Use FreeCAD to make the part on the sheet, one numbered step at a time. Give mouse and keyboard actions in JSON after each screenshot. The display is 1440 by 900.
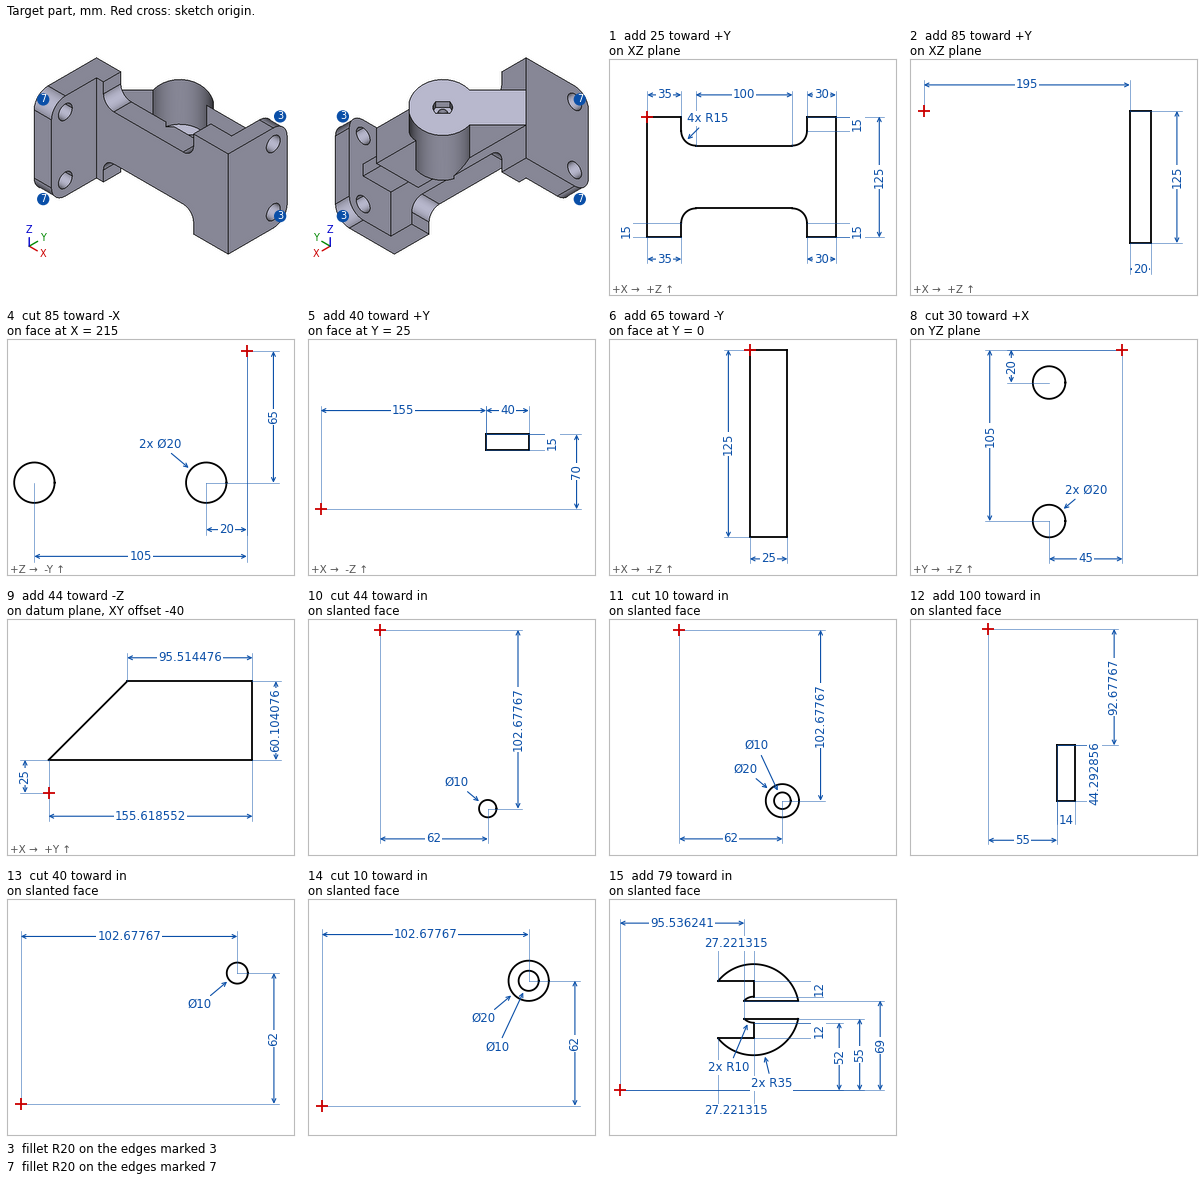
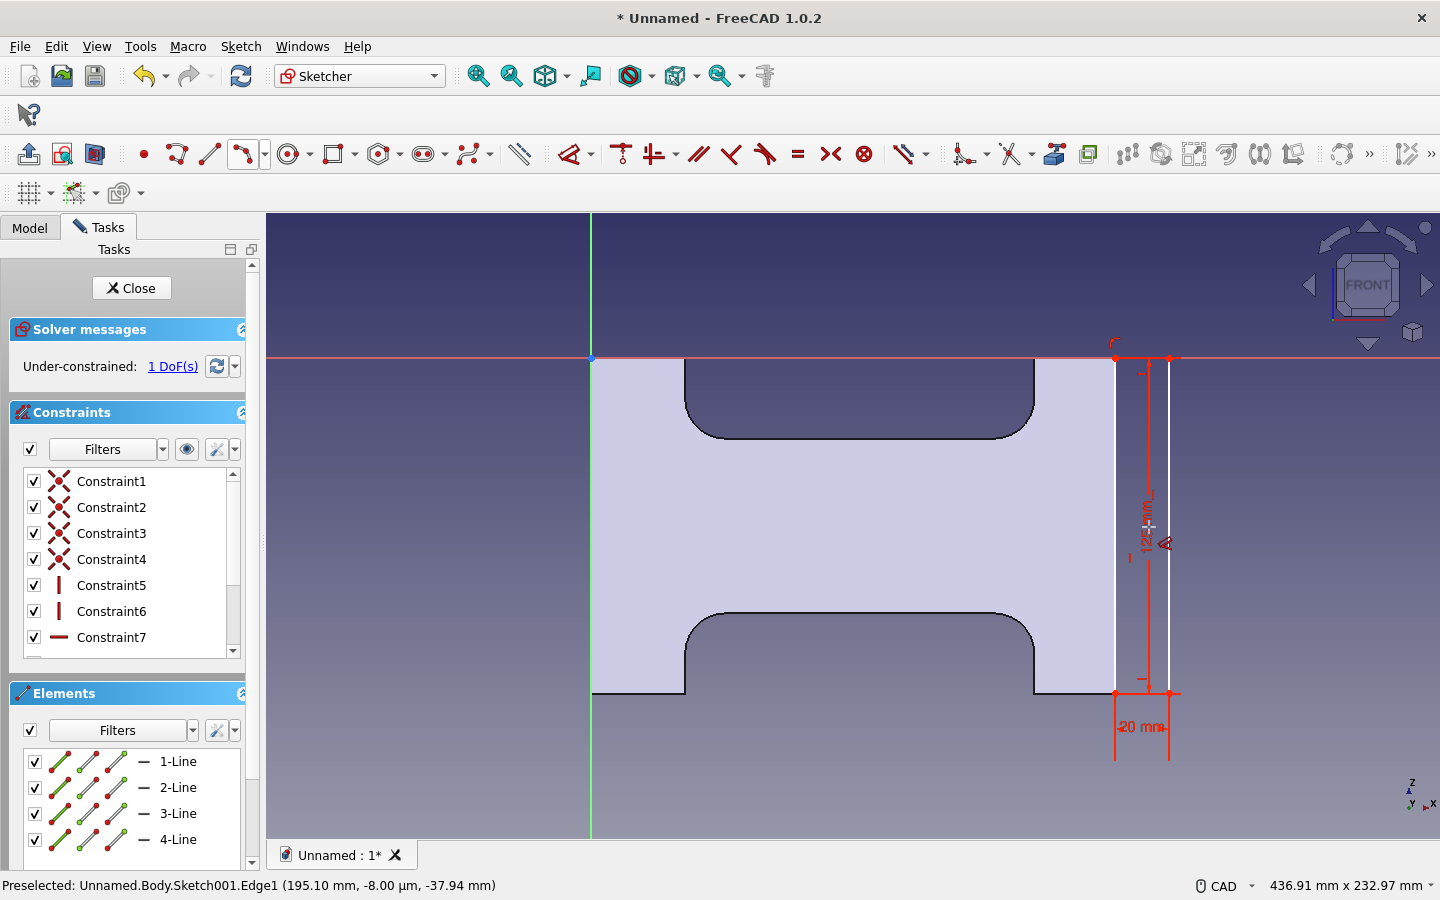
{"action": "left_click", "coordinate": [1115, 358]}
{"action": "left_click", "coordinate": [853, 324]}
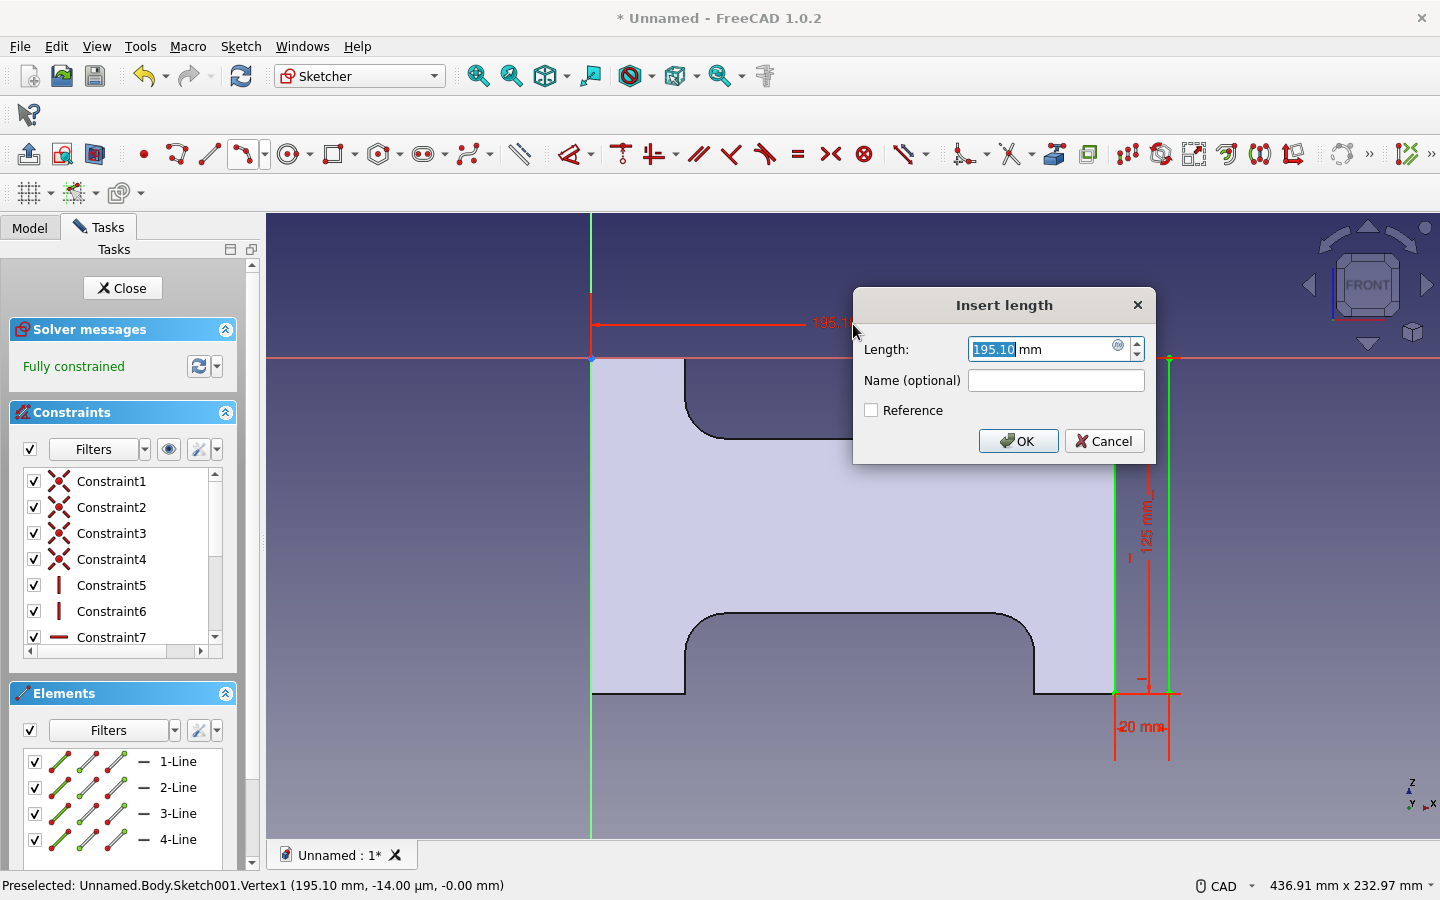
{"action": "type", "text": "195"}
{"action": "key", "text": "Return"}
{"action": "key", "text": "Escape"}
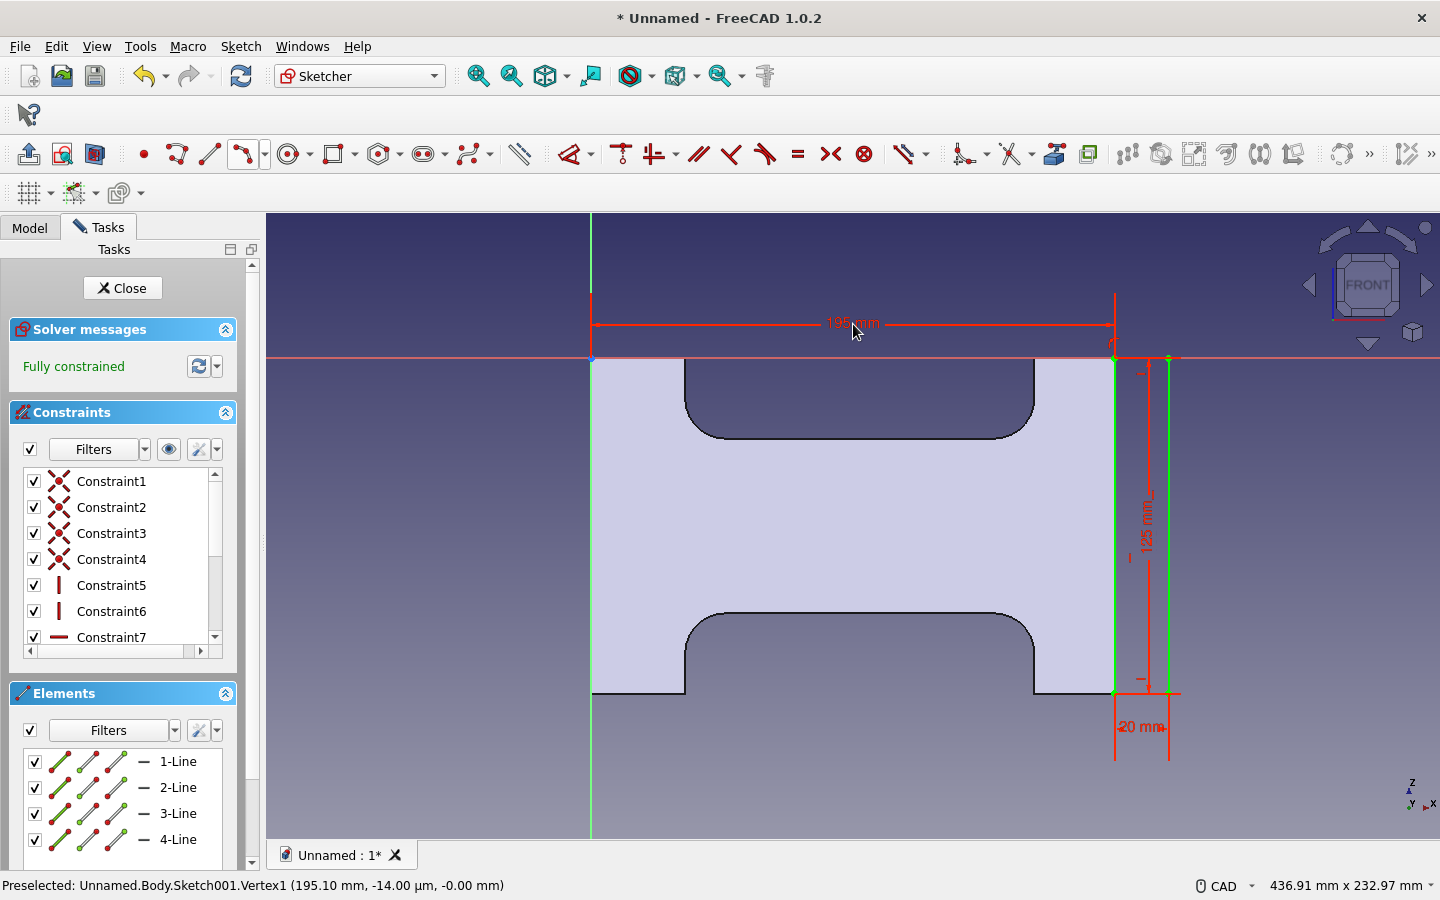
{"action": "left_click", "coordinate": [123, 288]}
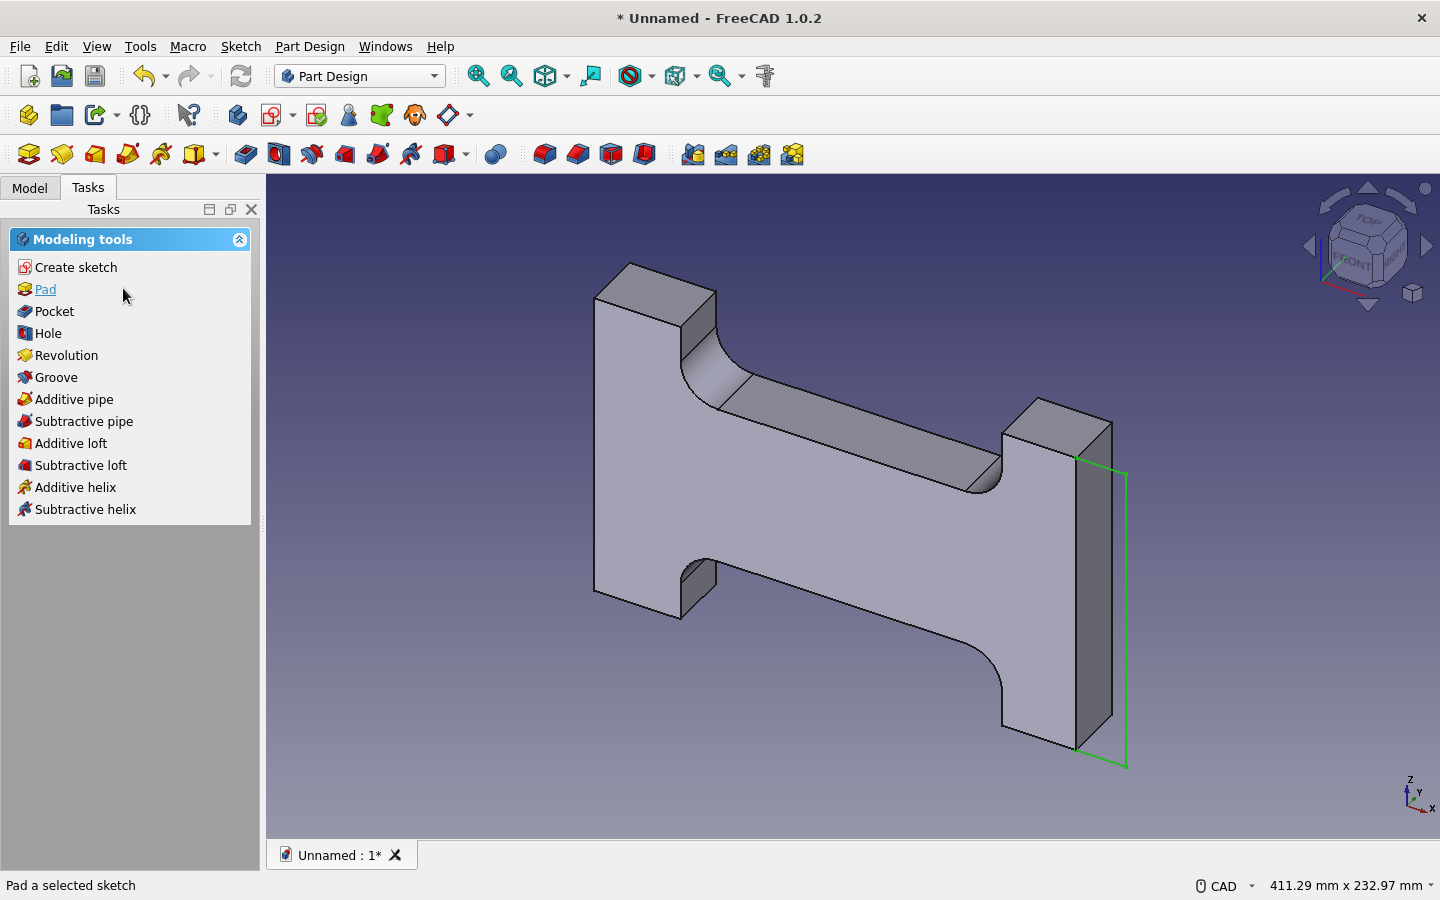
{"action": "left_click", "coordinate": [29, 154]}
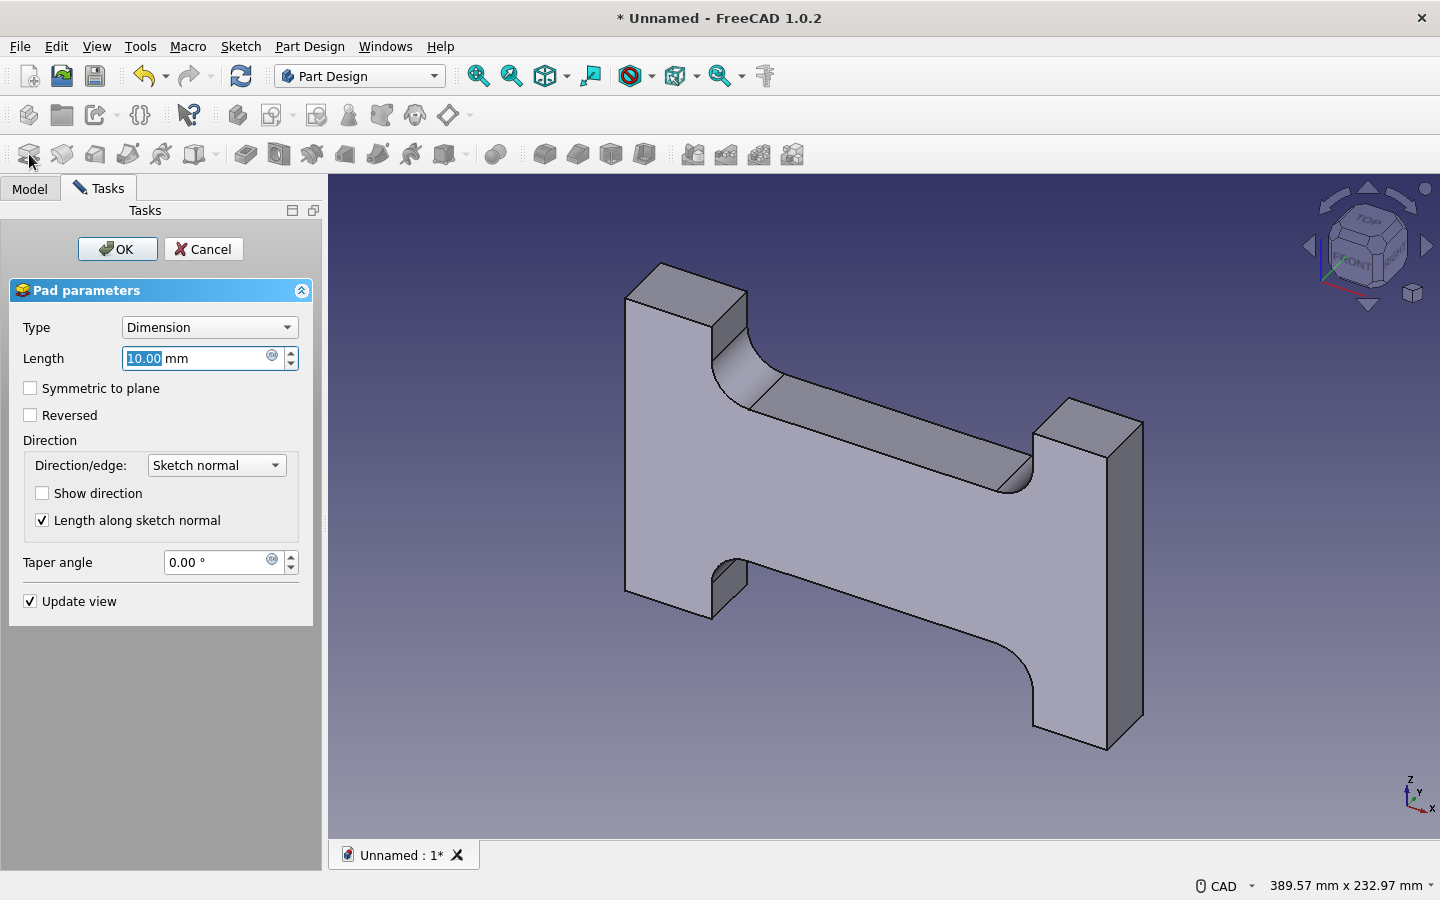
{"action": "type", "text": "85"}
{"action": "key", "text": "Tab"}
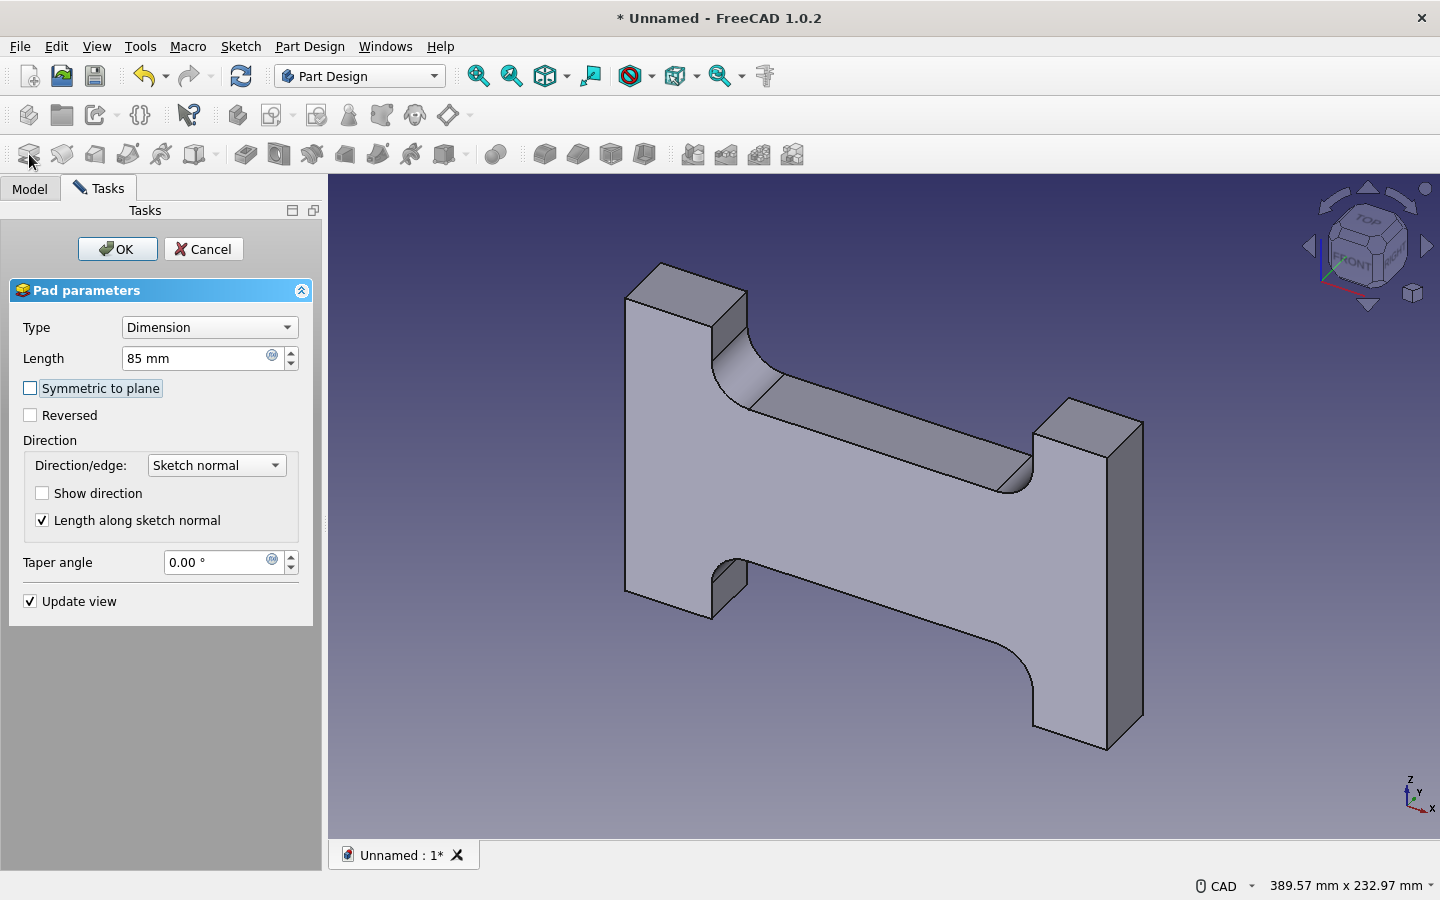
{"action": "left_click", "coordinate": [31, 415]}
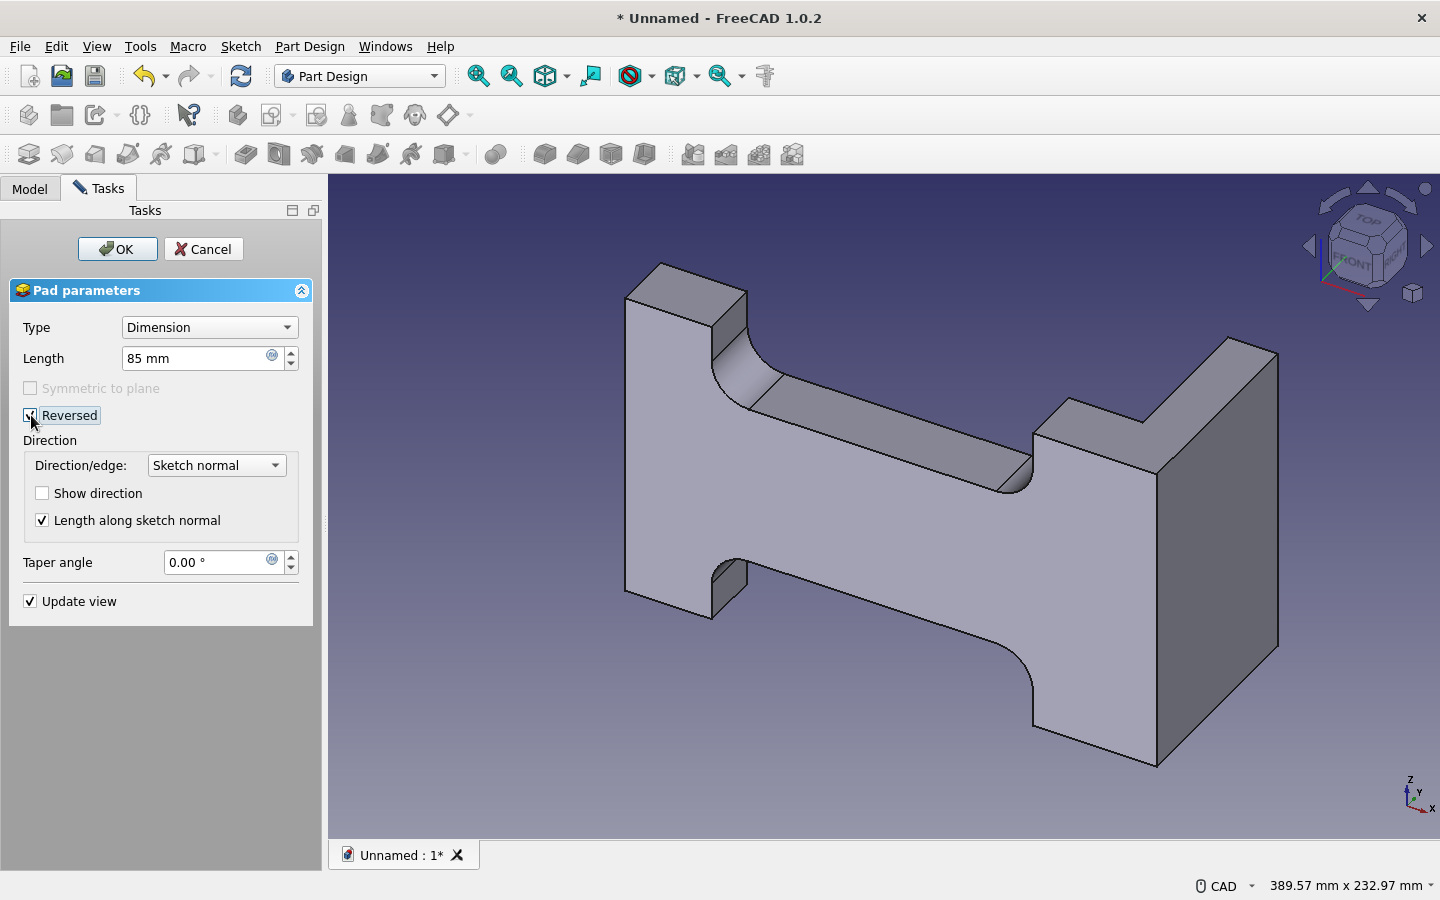
{"action": "left_click", "coordinate": [118, 249]}